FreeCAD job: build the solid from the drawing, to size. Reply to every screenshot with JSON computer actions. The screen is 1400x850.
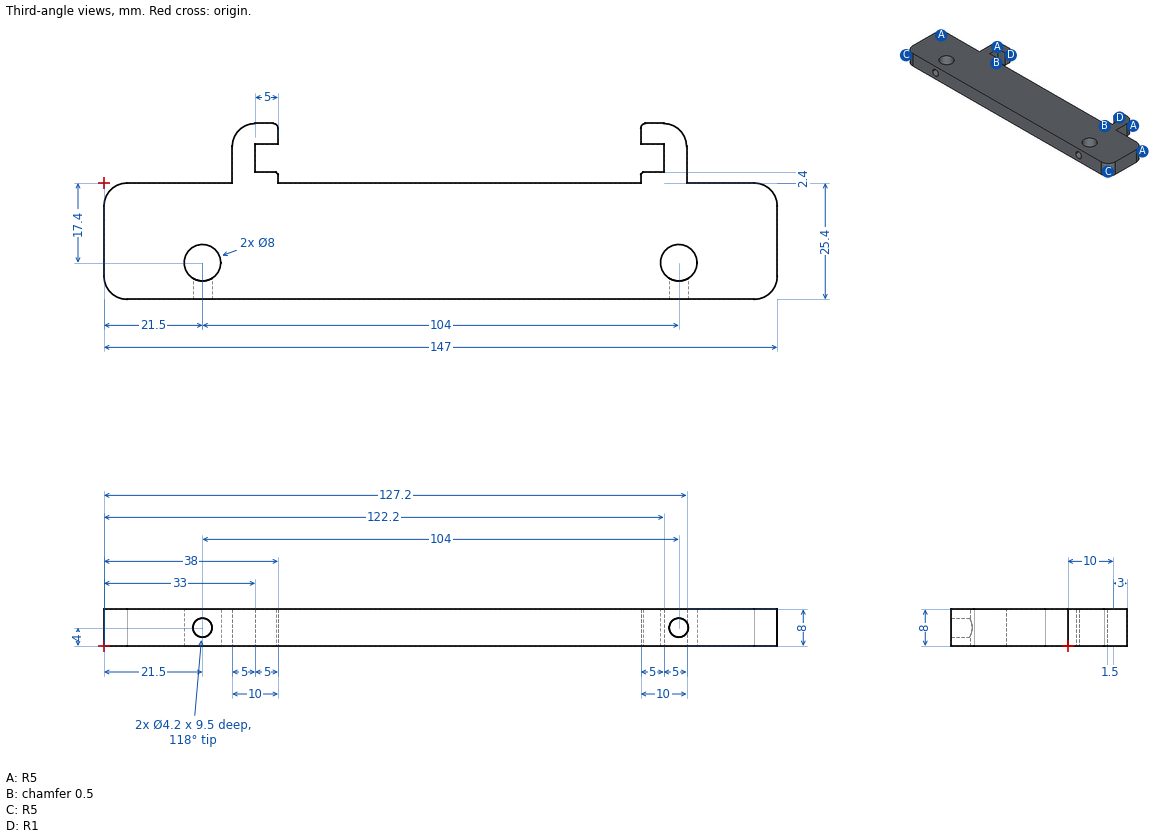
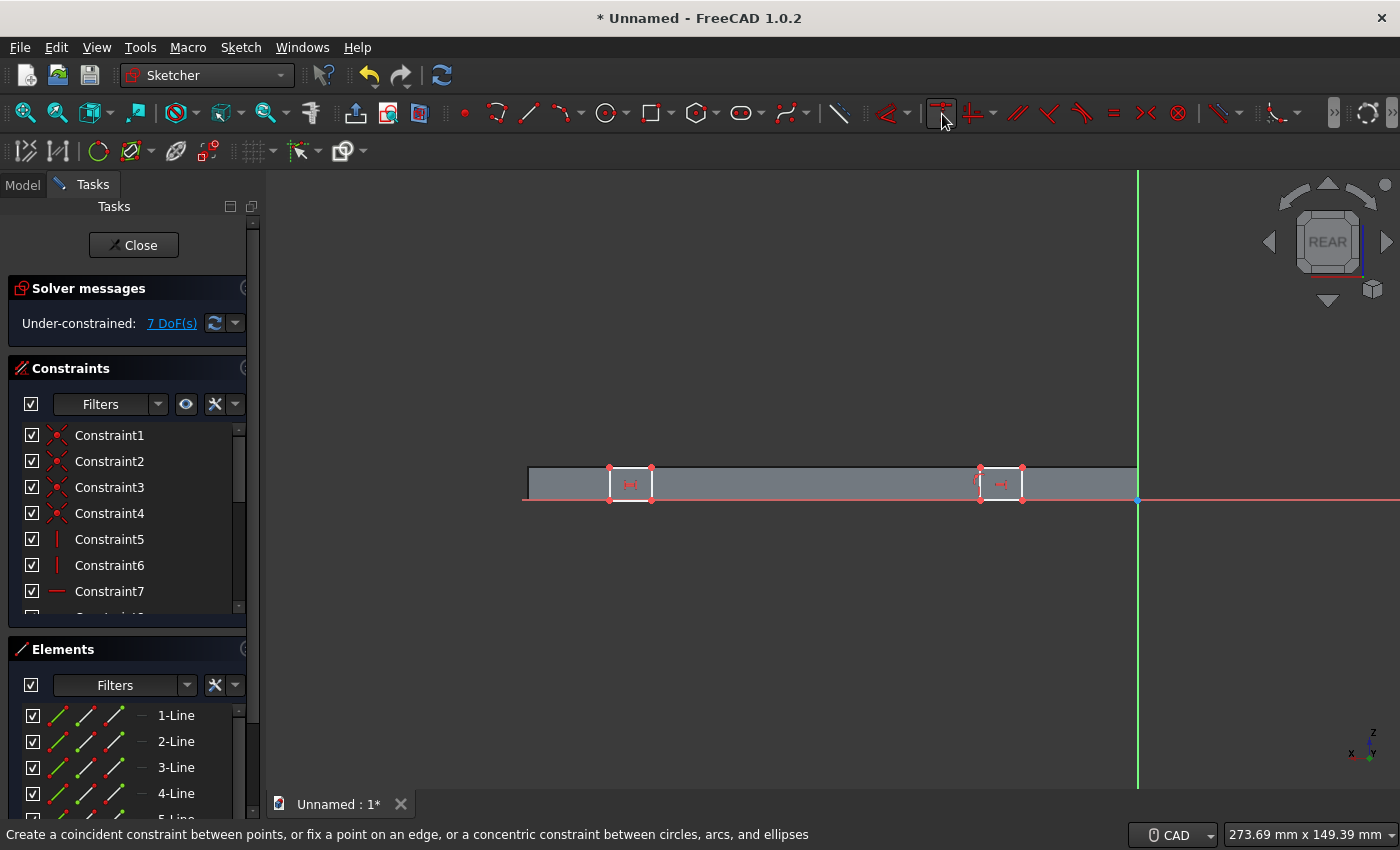
{"action": "left_click", "coordinate": [610, 501]}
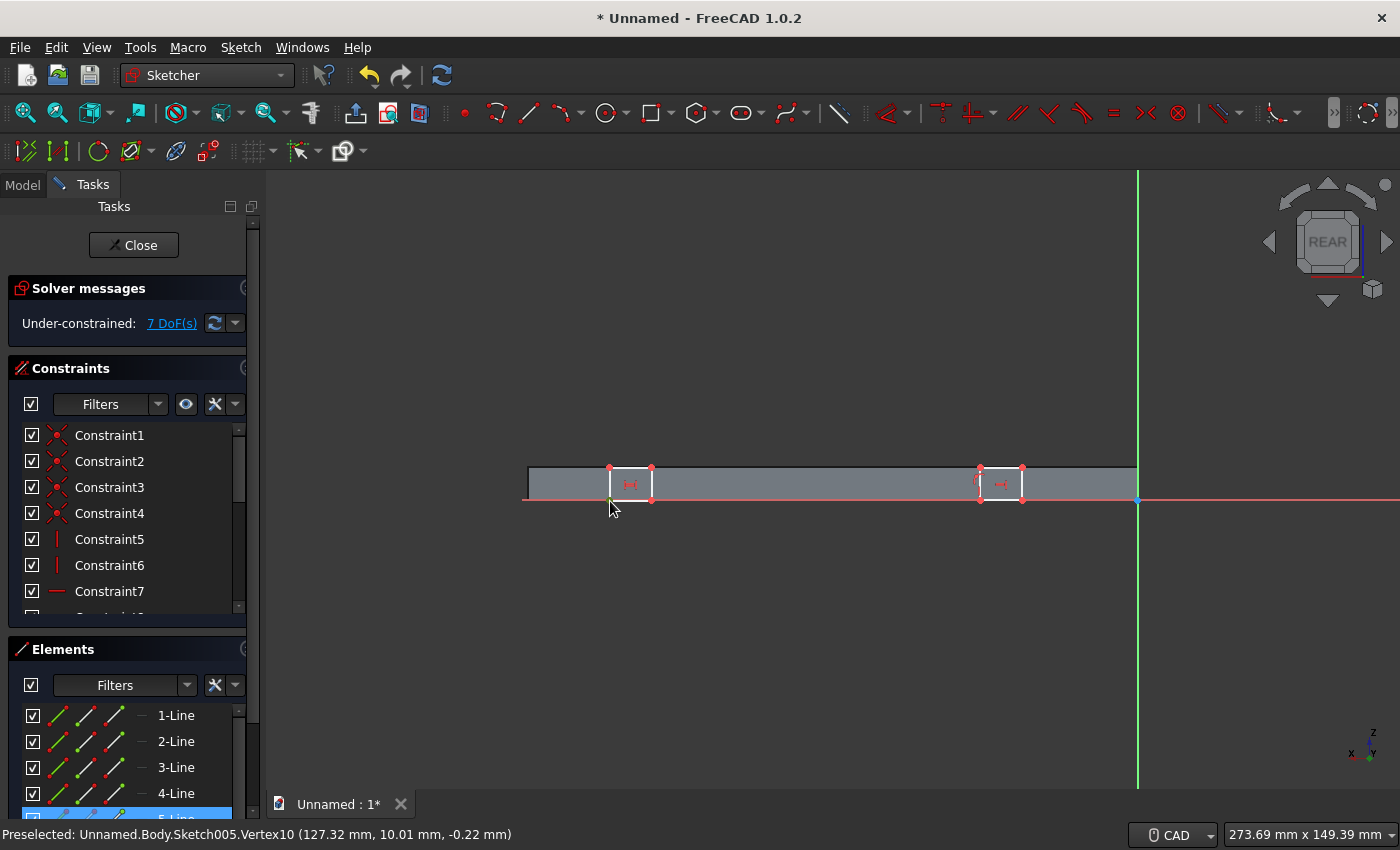
{"action": "left_click", "coordinate": [563, 500]}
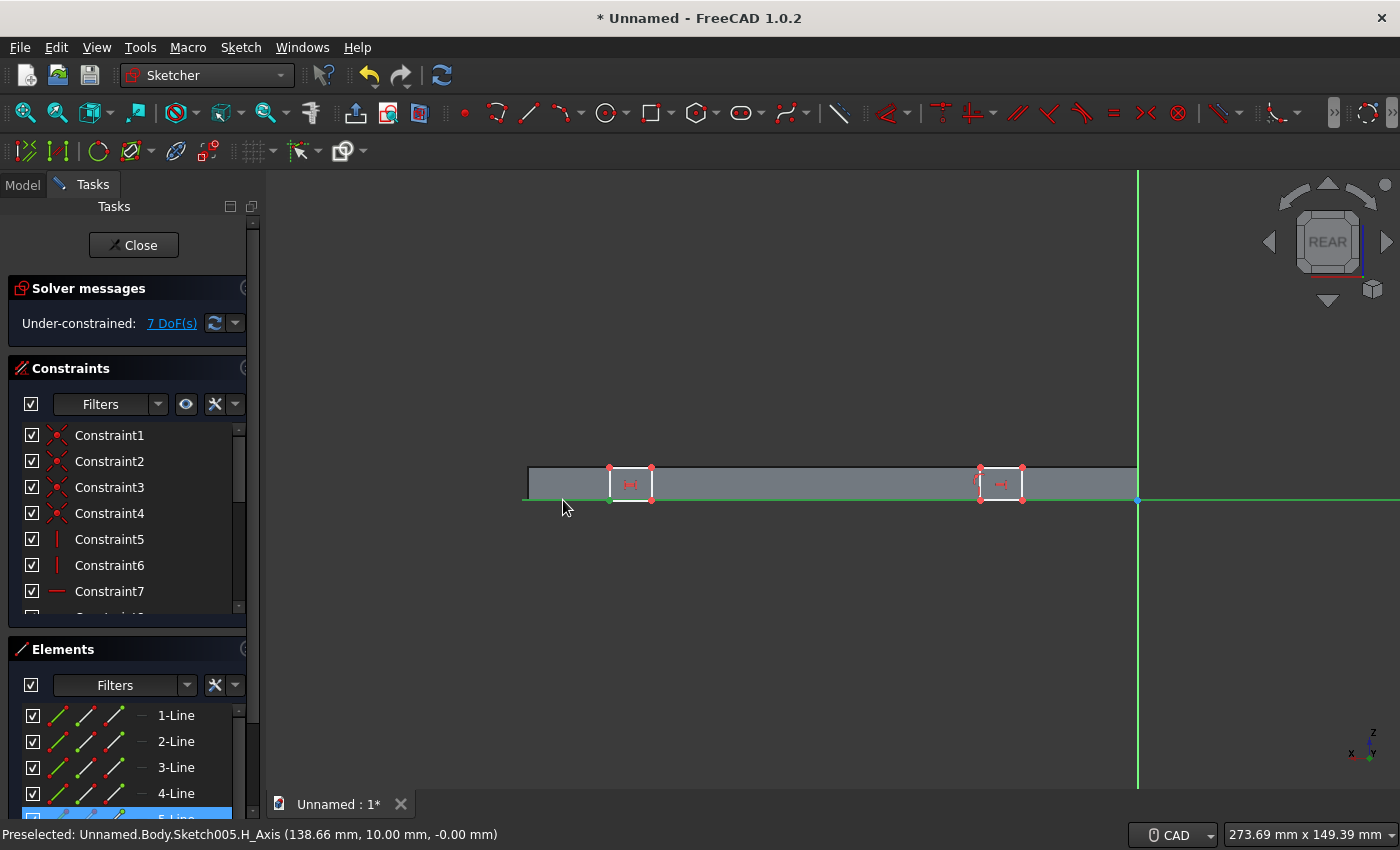
{"action": "left_click", "coordinate": [942, 114]}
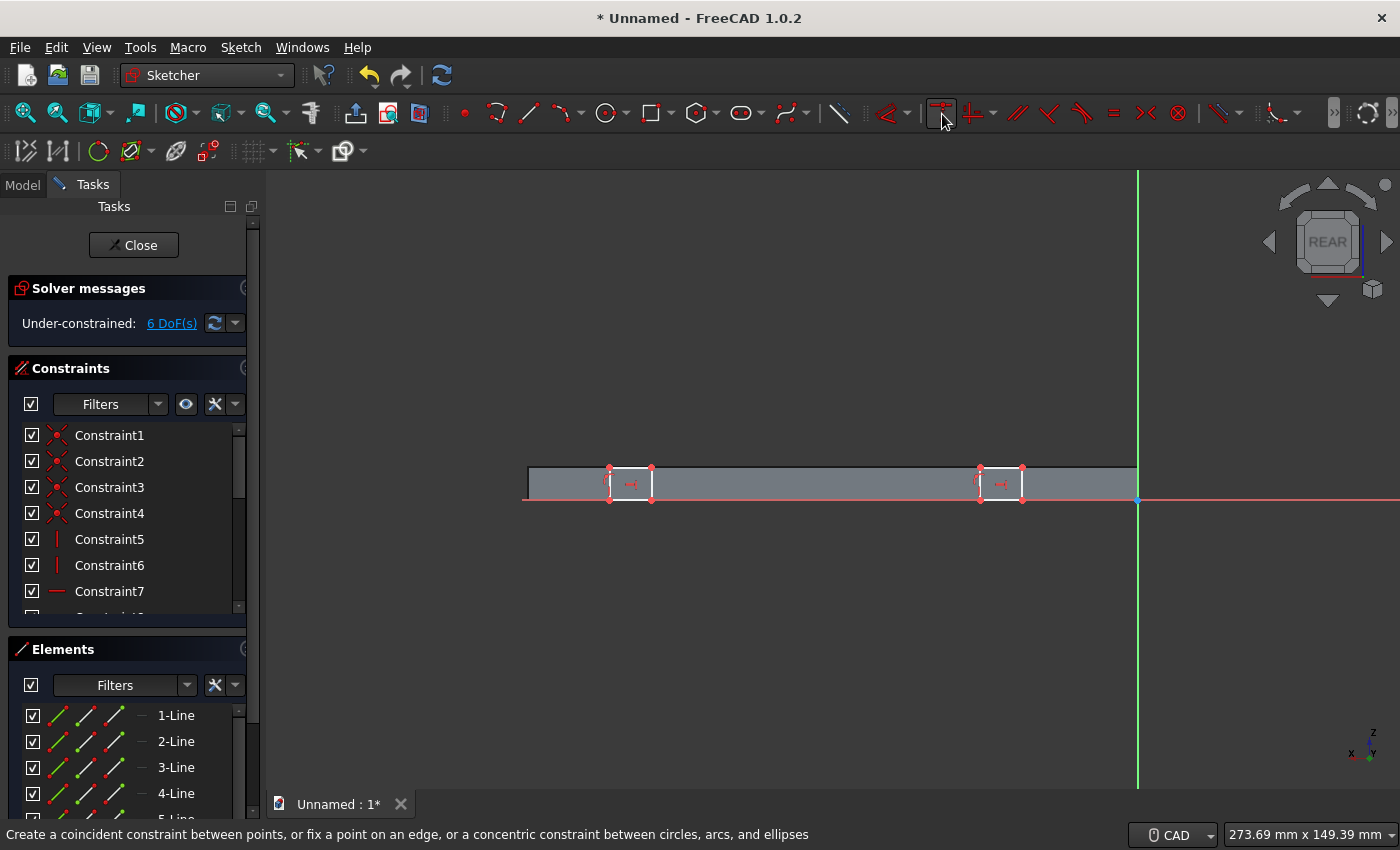
{"action": "left_click", "coordinate": [886, 114]}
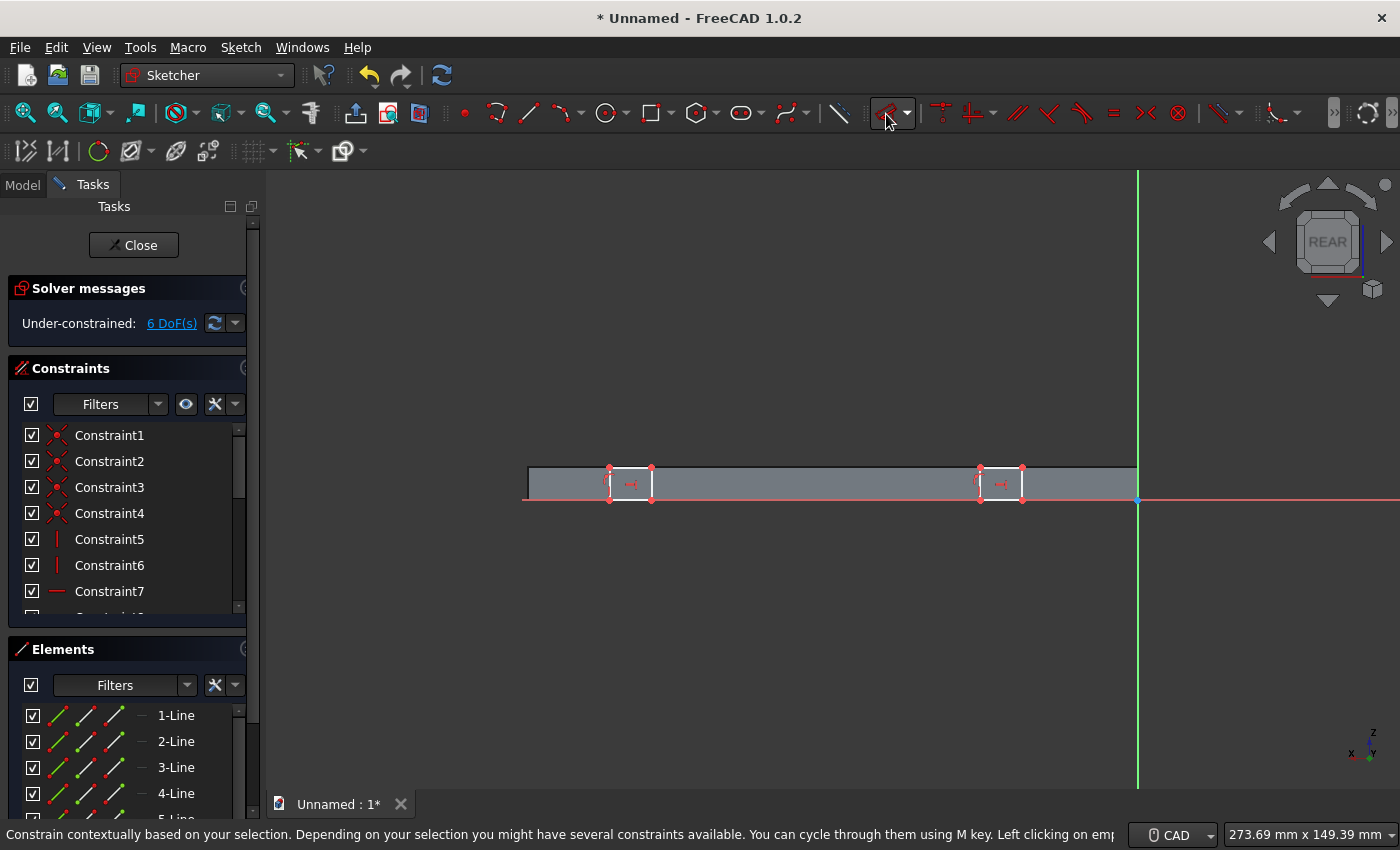
{"action": "scroll", "coordinate": [980, 478], "scroll_direction": "up", "scroll_amount": 2}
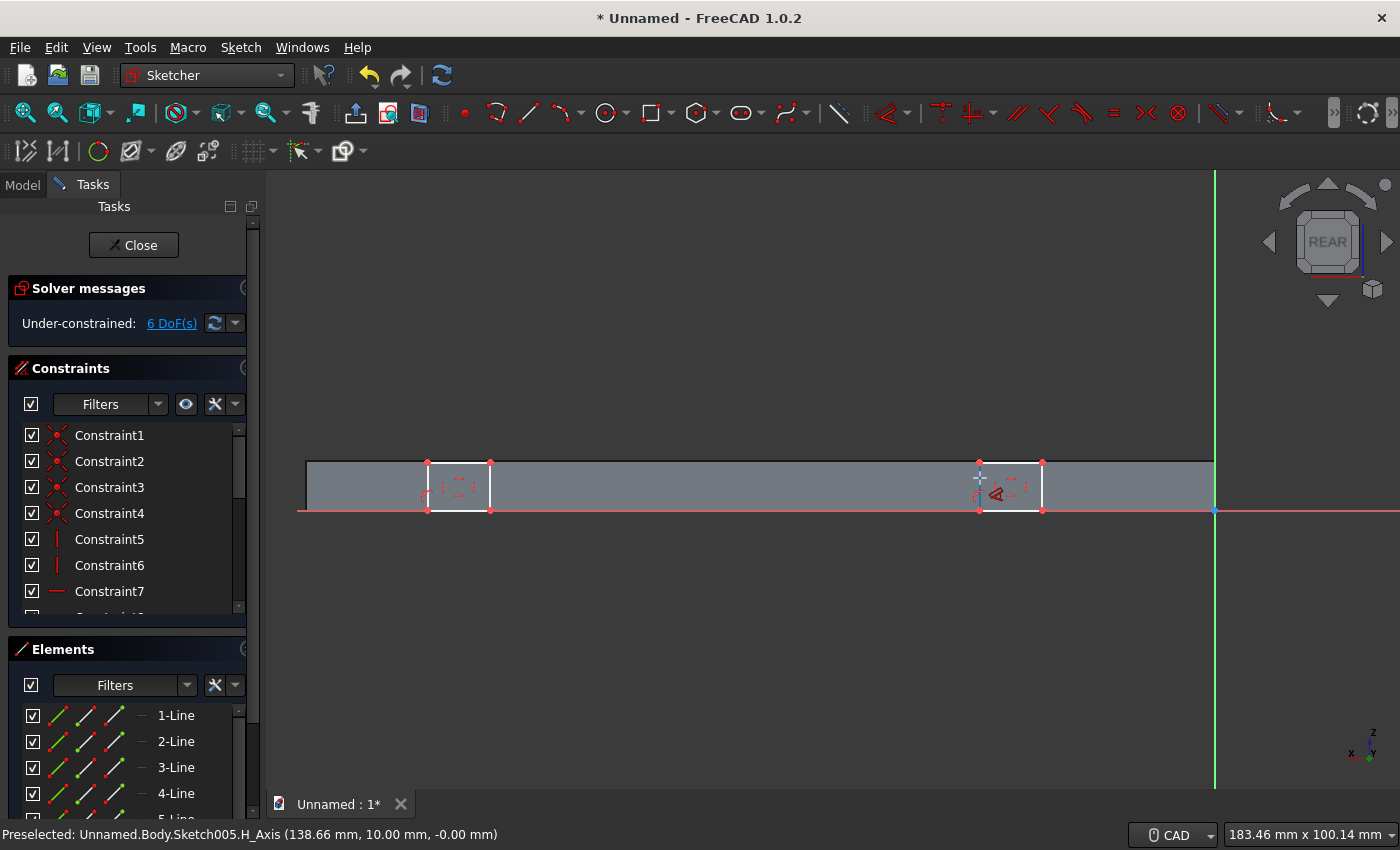
{"action": "left_click", "coordinate": [980, 477]}
{"action": "left_click", "coordinate": [1014, 487]}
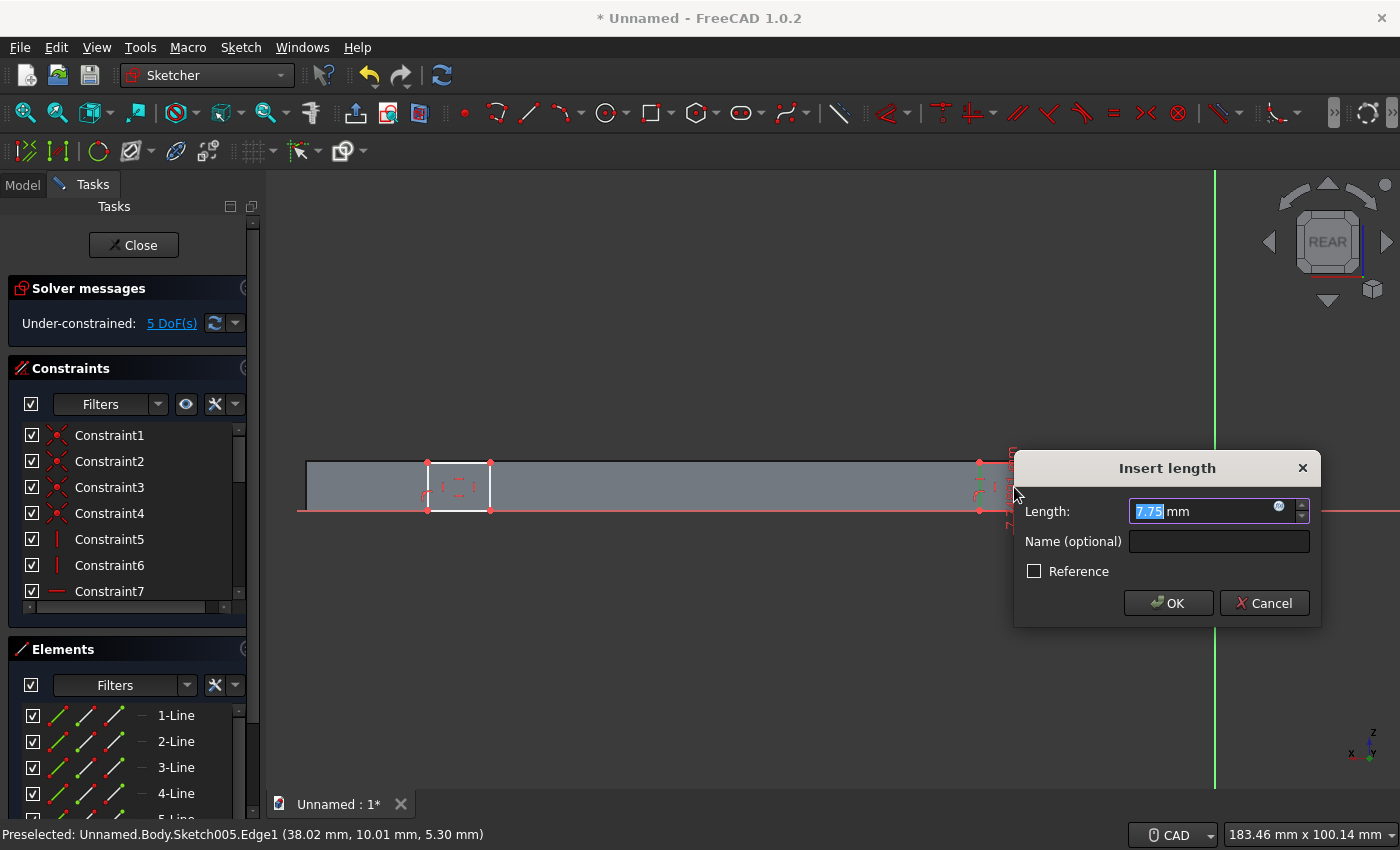
{"action": "type", "text": "8"}
{"action": "key", "text": "Return"}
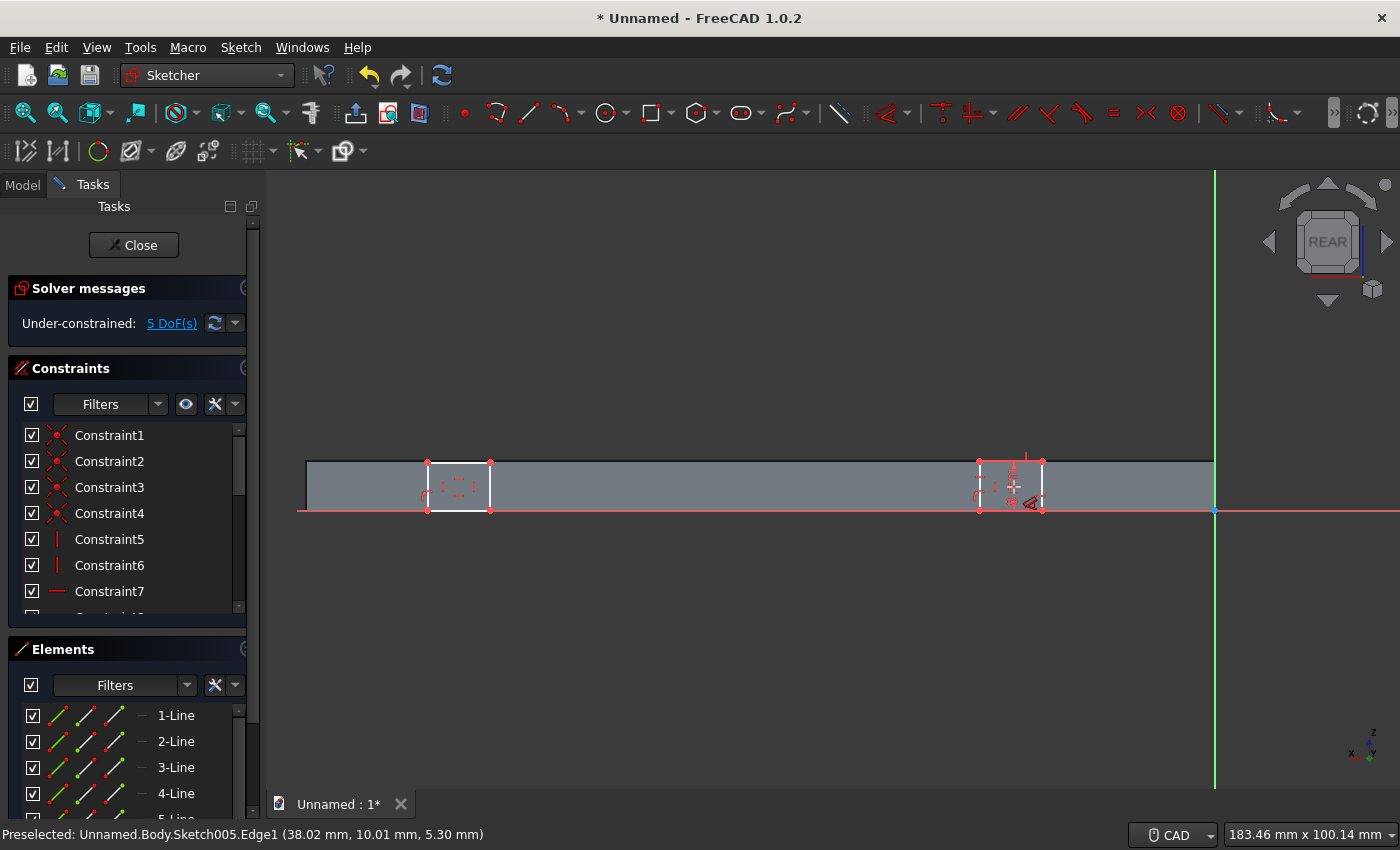
{"action": "left_click", "coordinate": [428, 477]}
{"action": "left_click", "coordinate": [394, 487]}